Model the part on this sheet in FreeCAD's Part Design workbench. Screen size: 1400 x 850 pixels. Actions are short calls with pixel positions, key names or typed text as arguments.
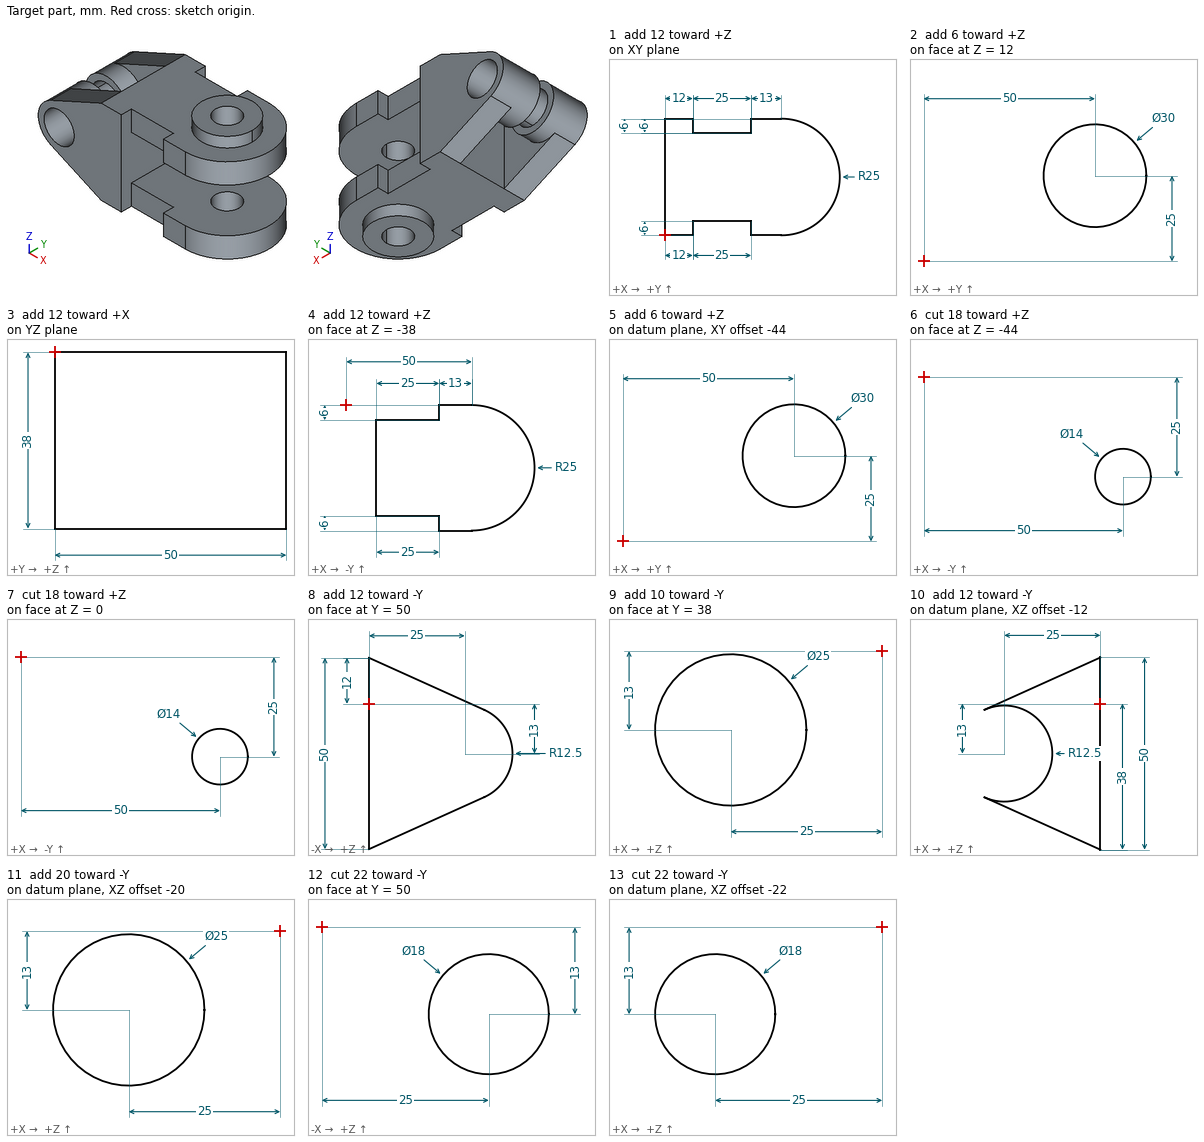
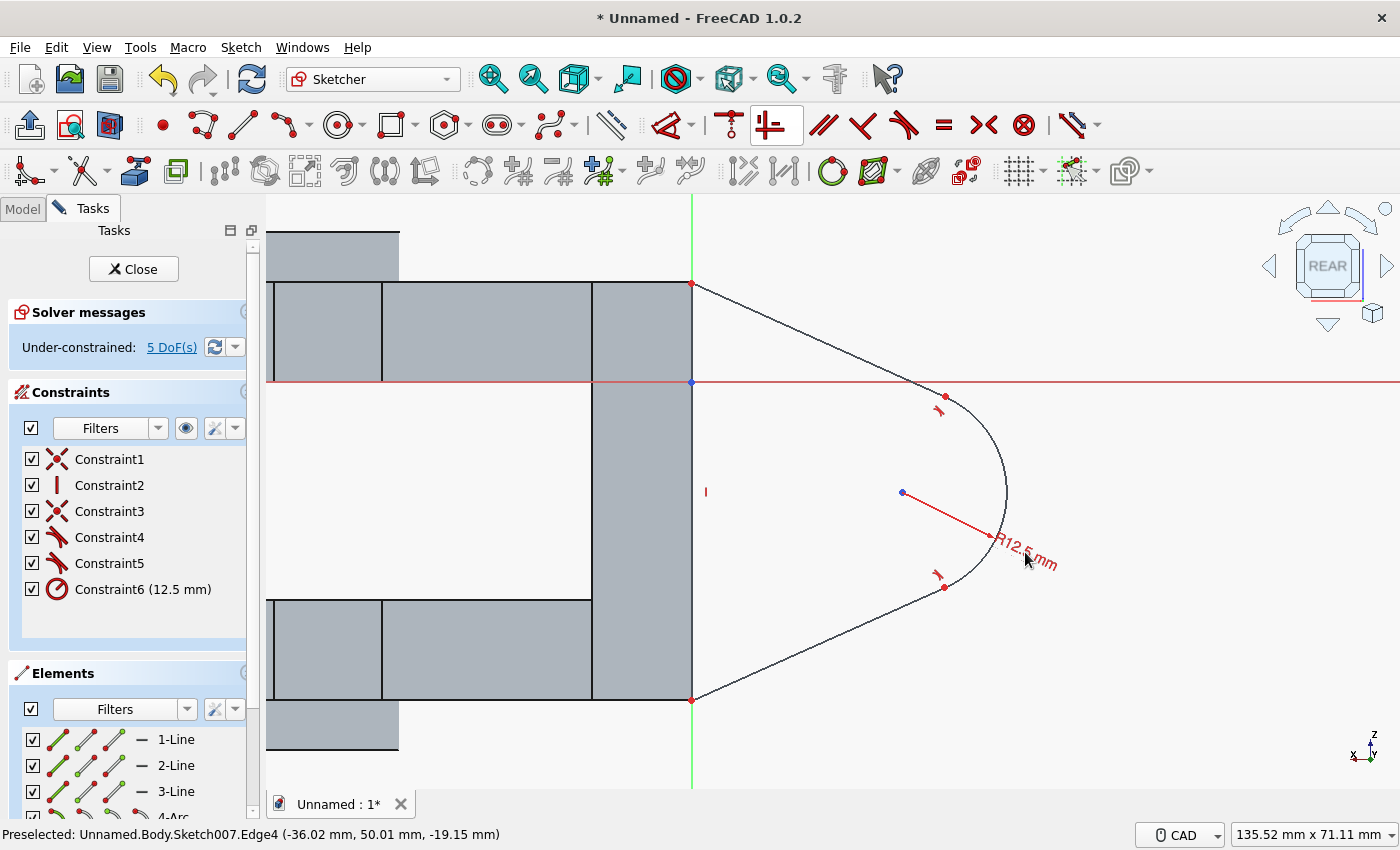
click(692, 283)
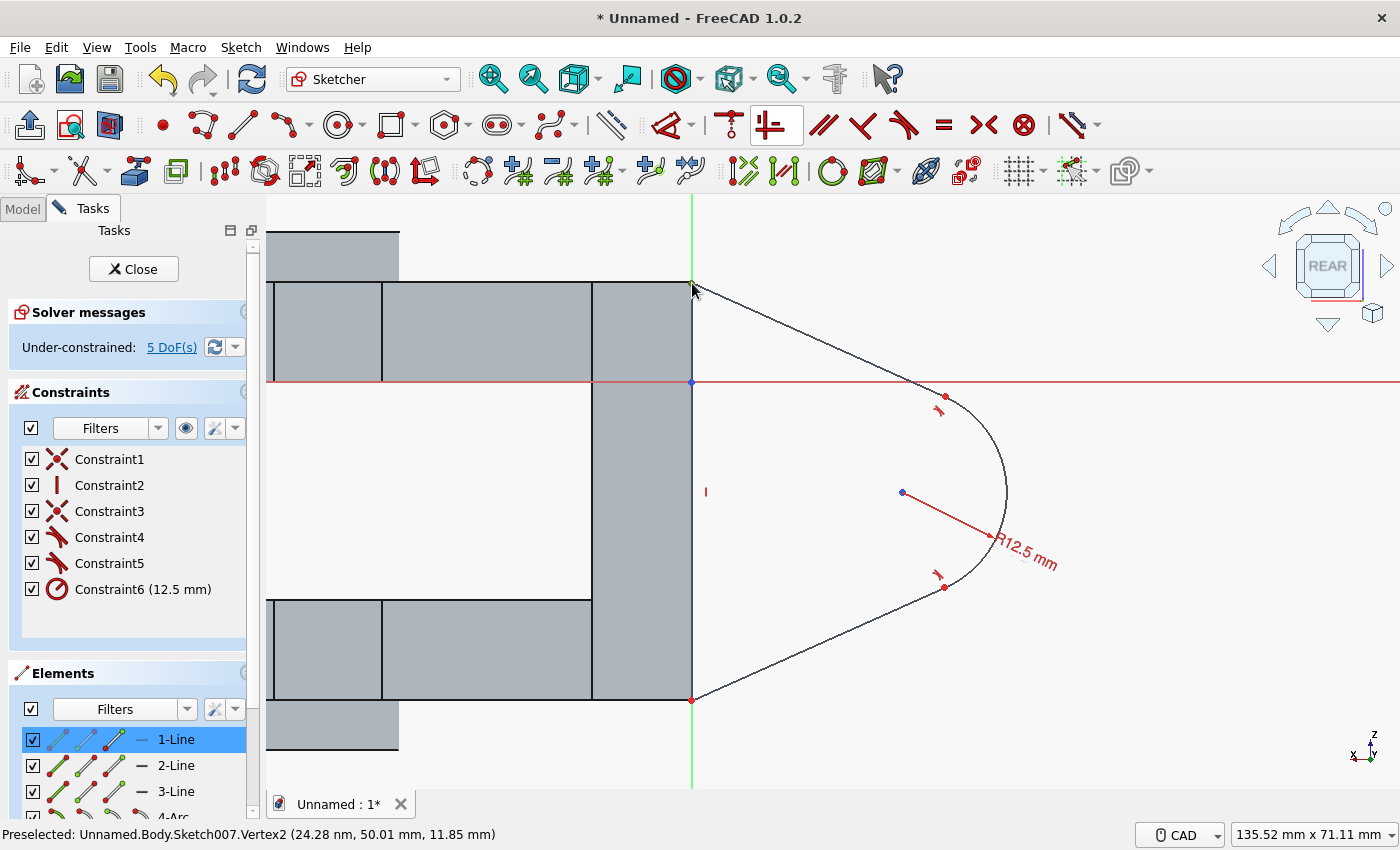
click(692, 261)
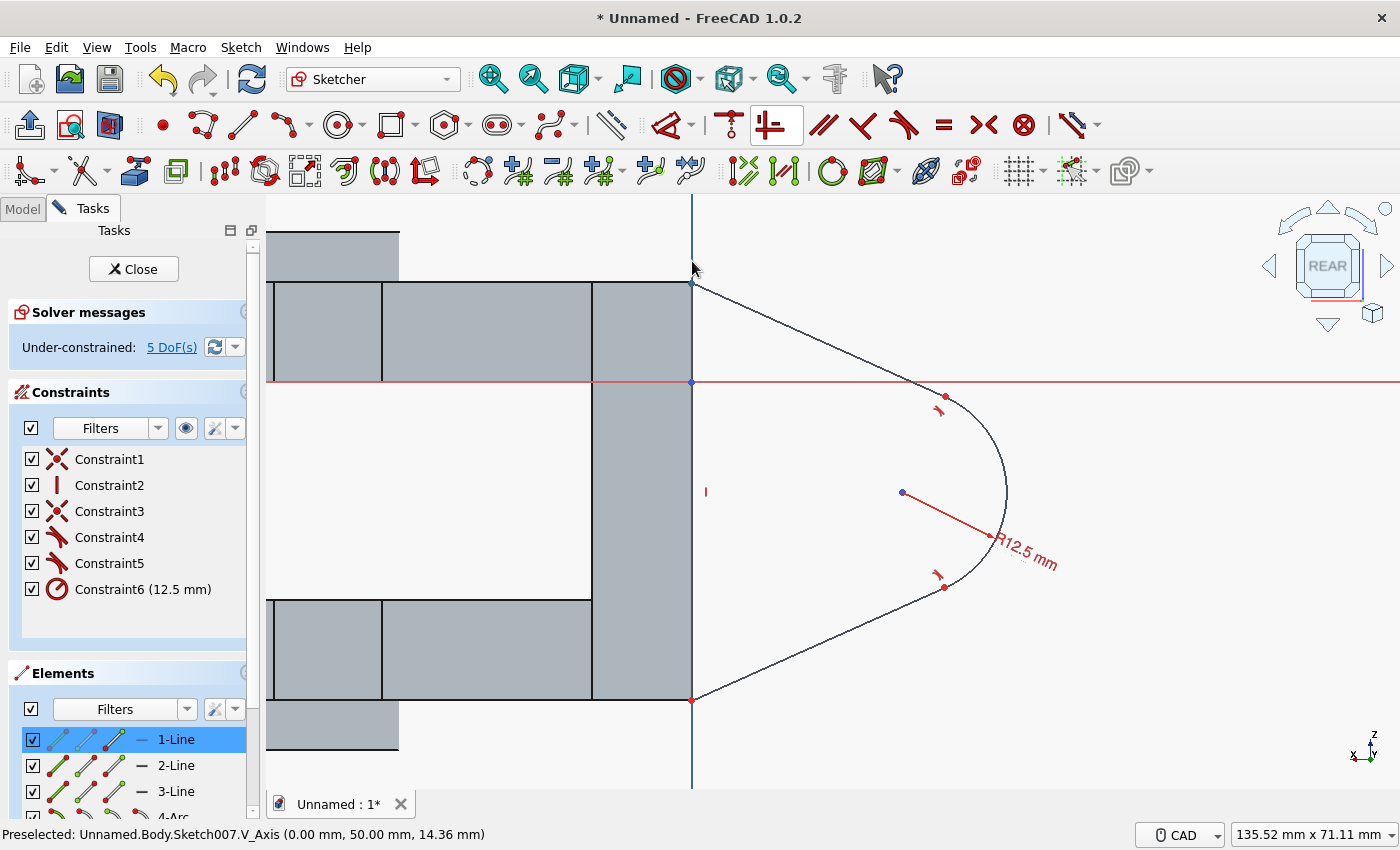
key(c)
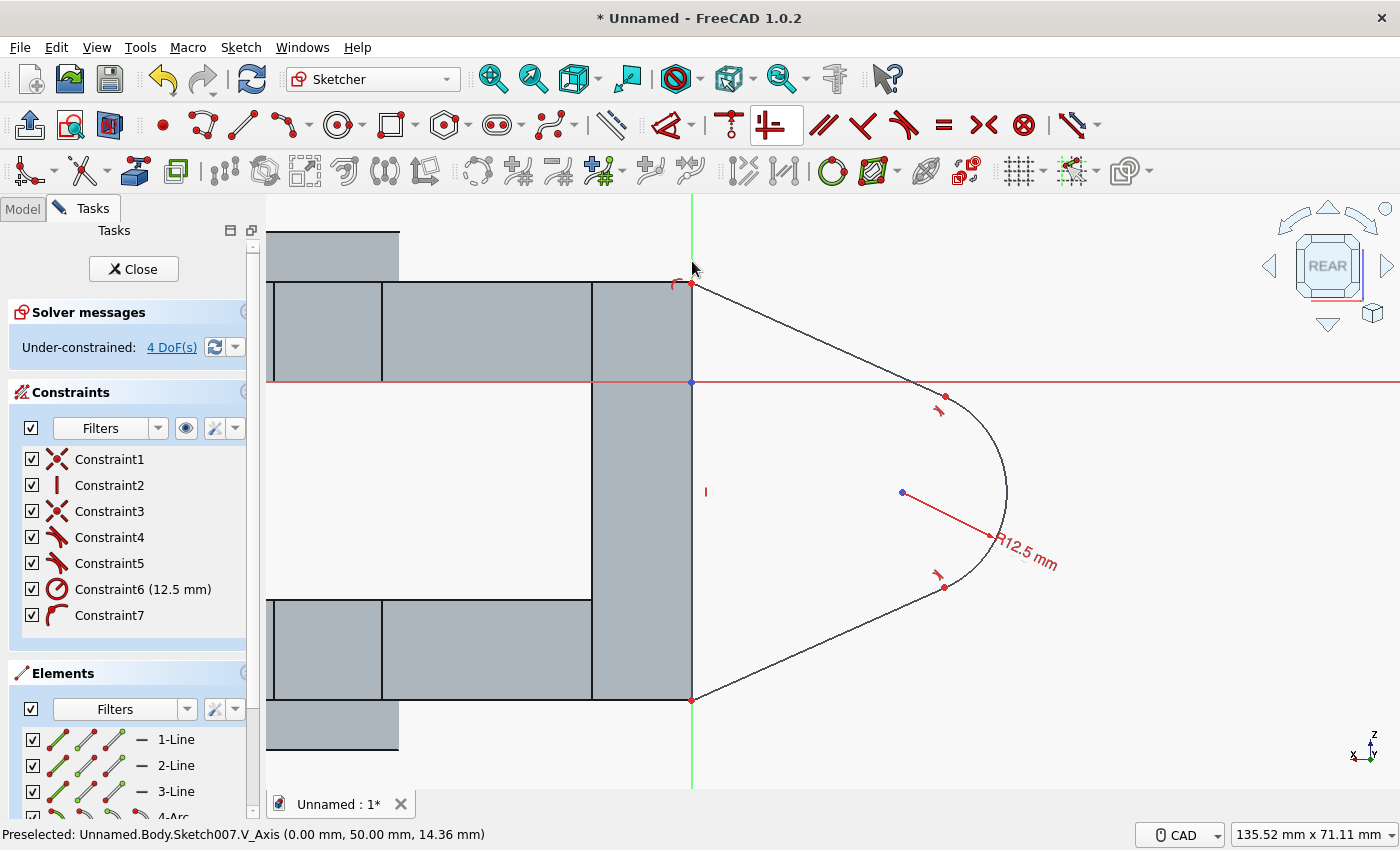
key(d)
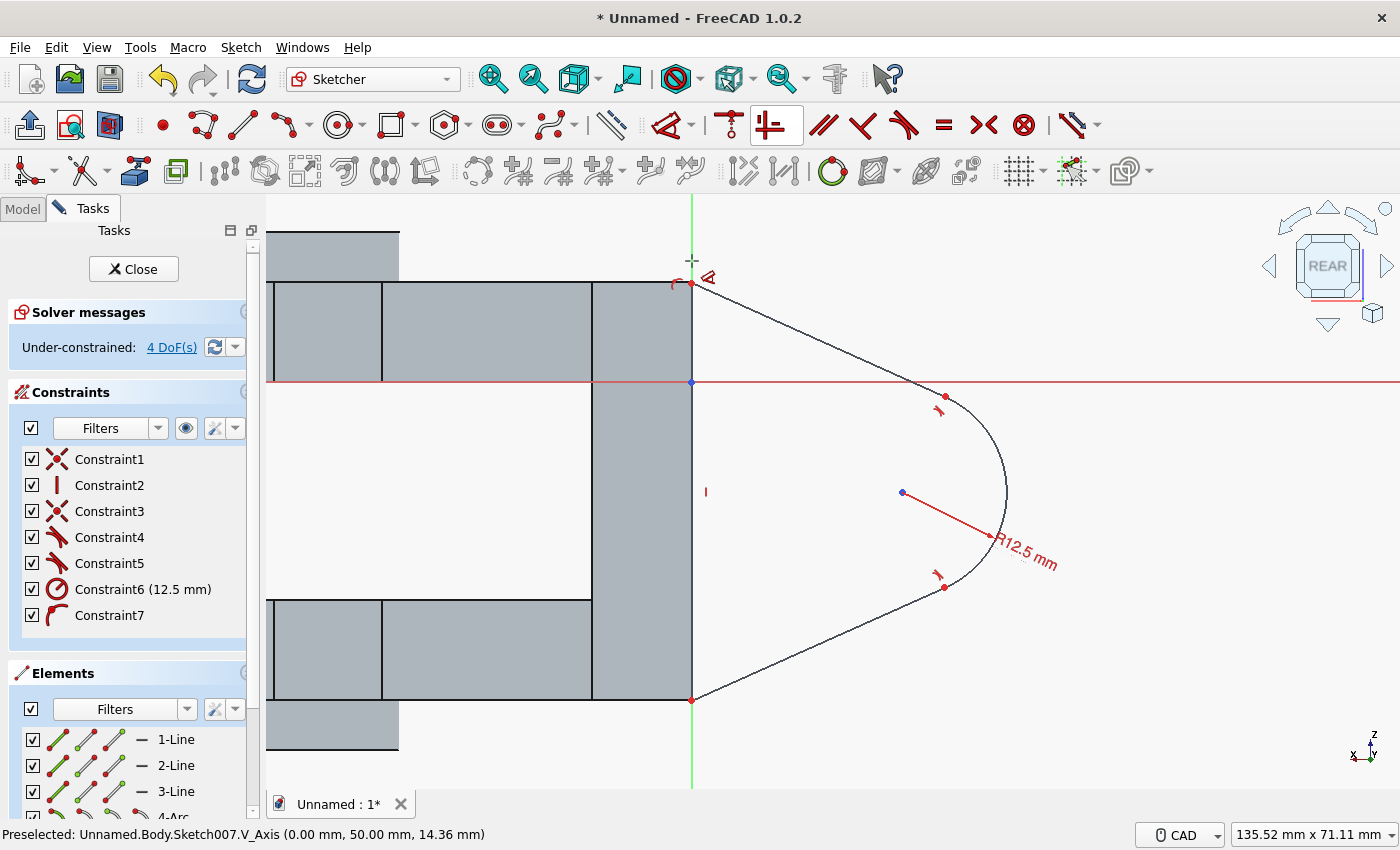
click(692, 408)
click(658, 492)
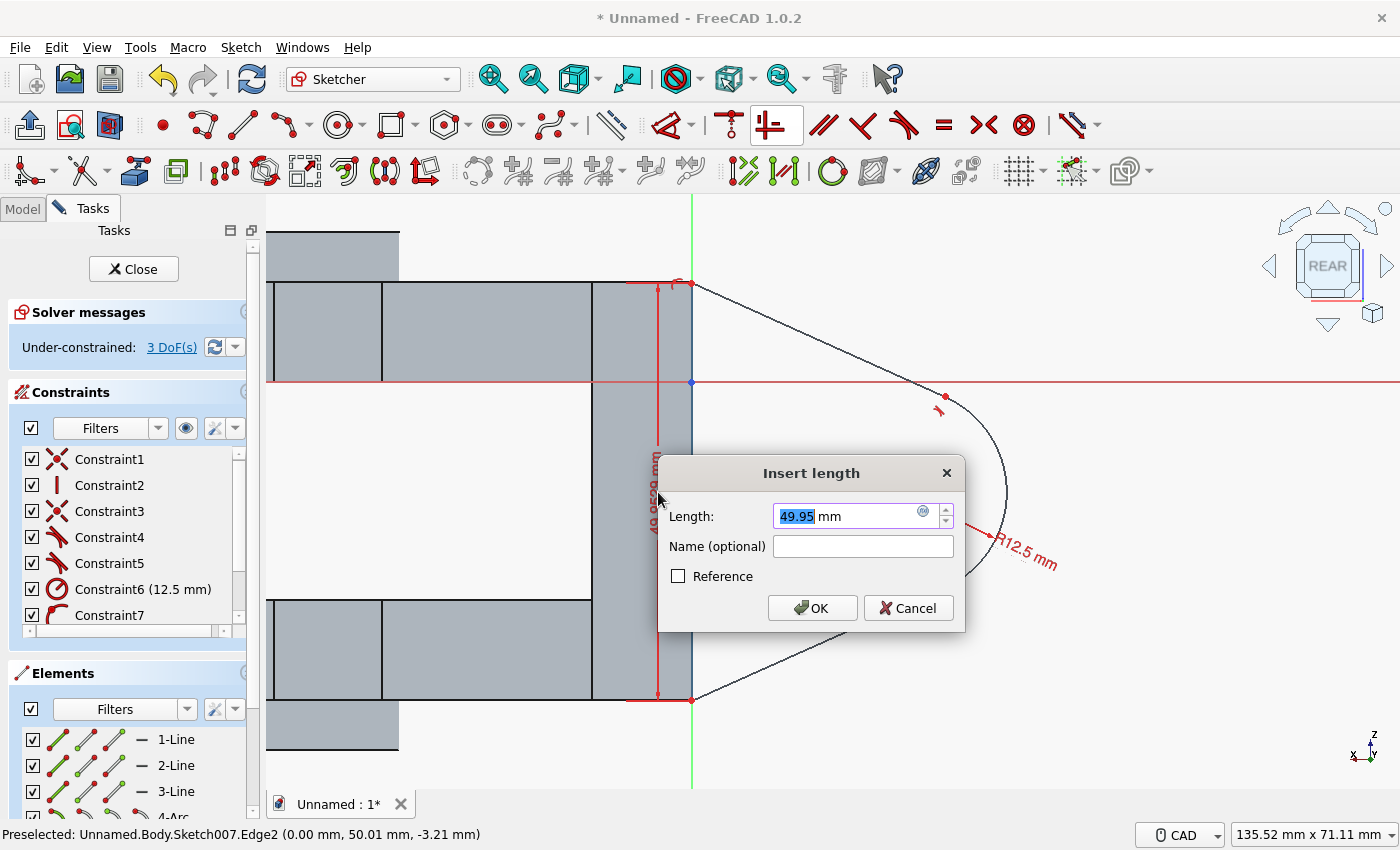
text(50)
key(Return)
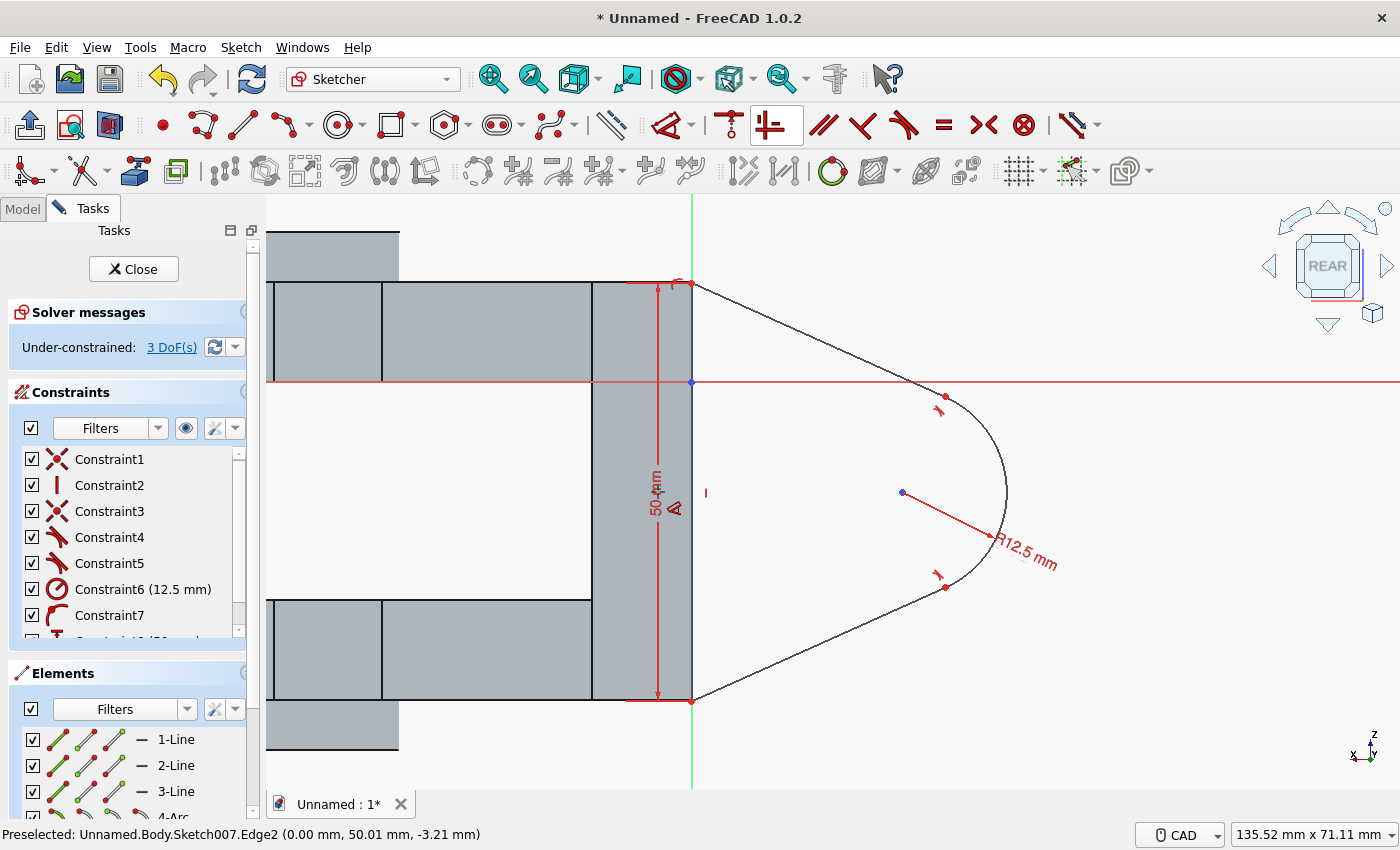
click(692, 283)
click(658, 333)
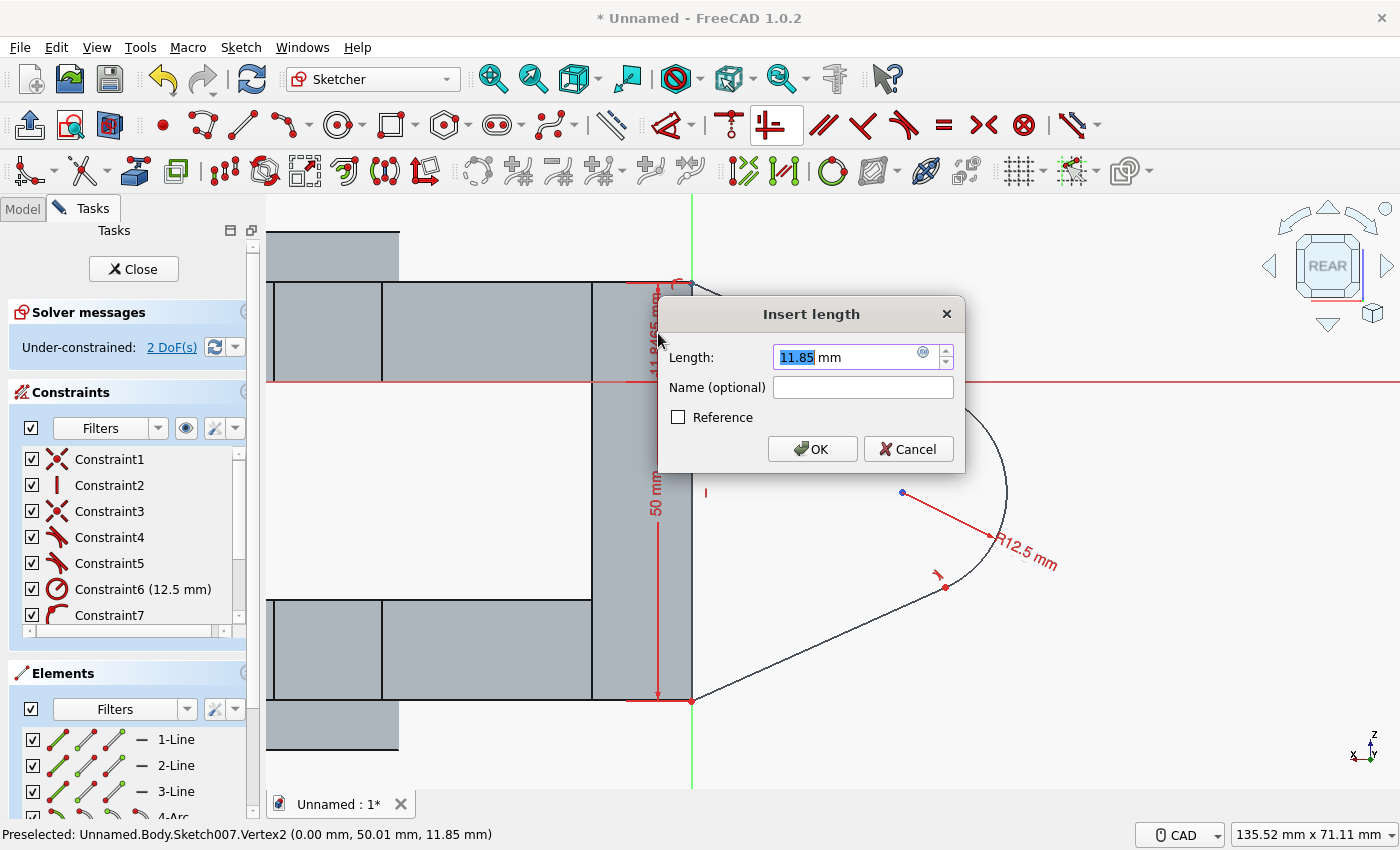
text(12)
key(Return)